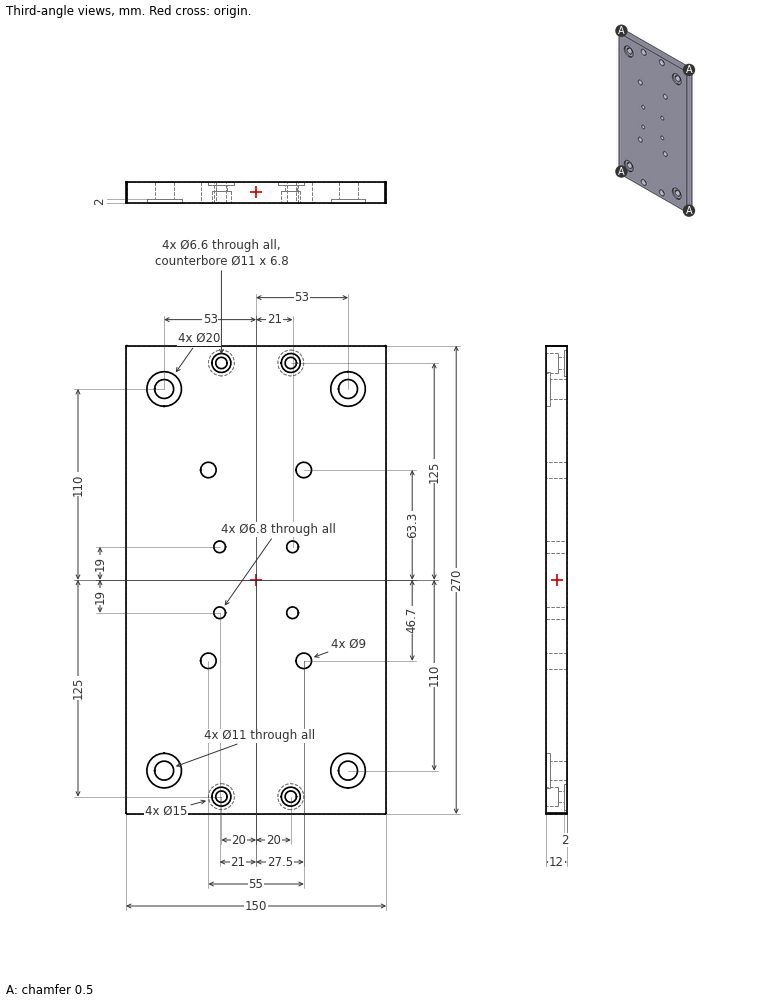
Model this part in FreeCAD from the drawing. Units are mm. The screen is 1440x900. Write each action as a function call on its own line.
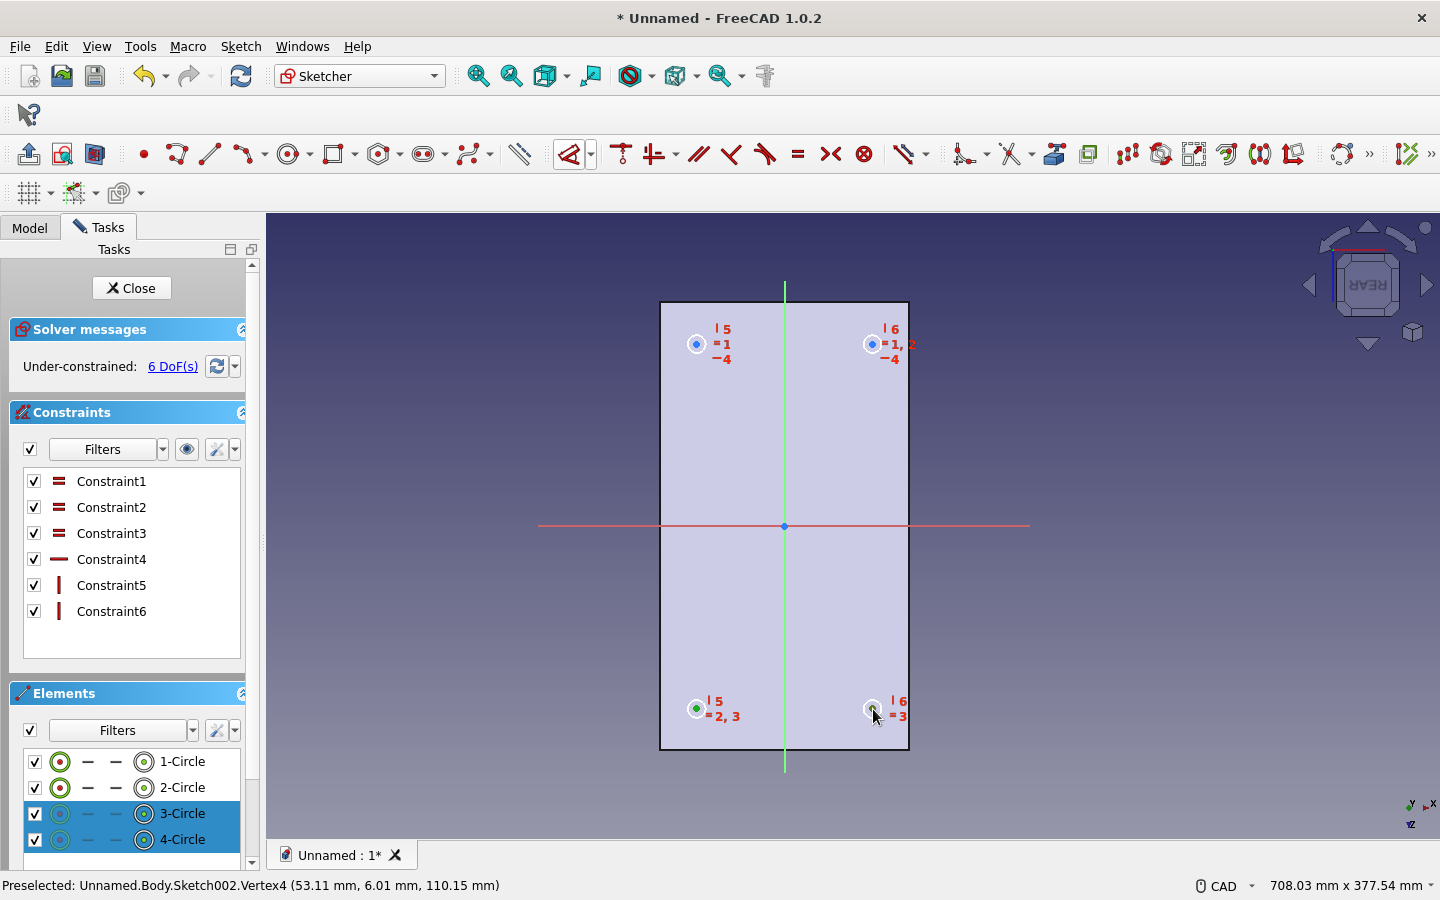
click(676, 154)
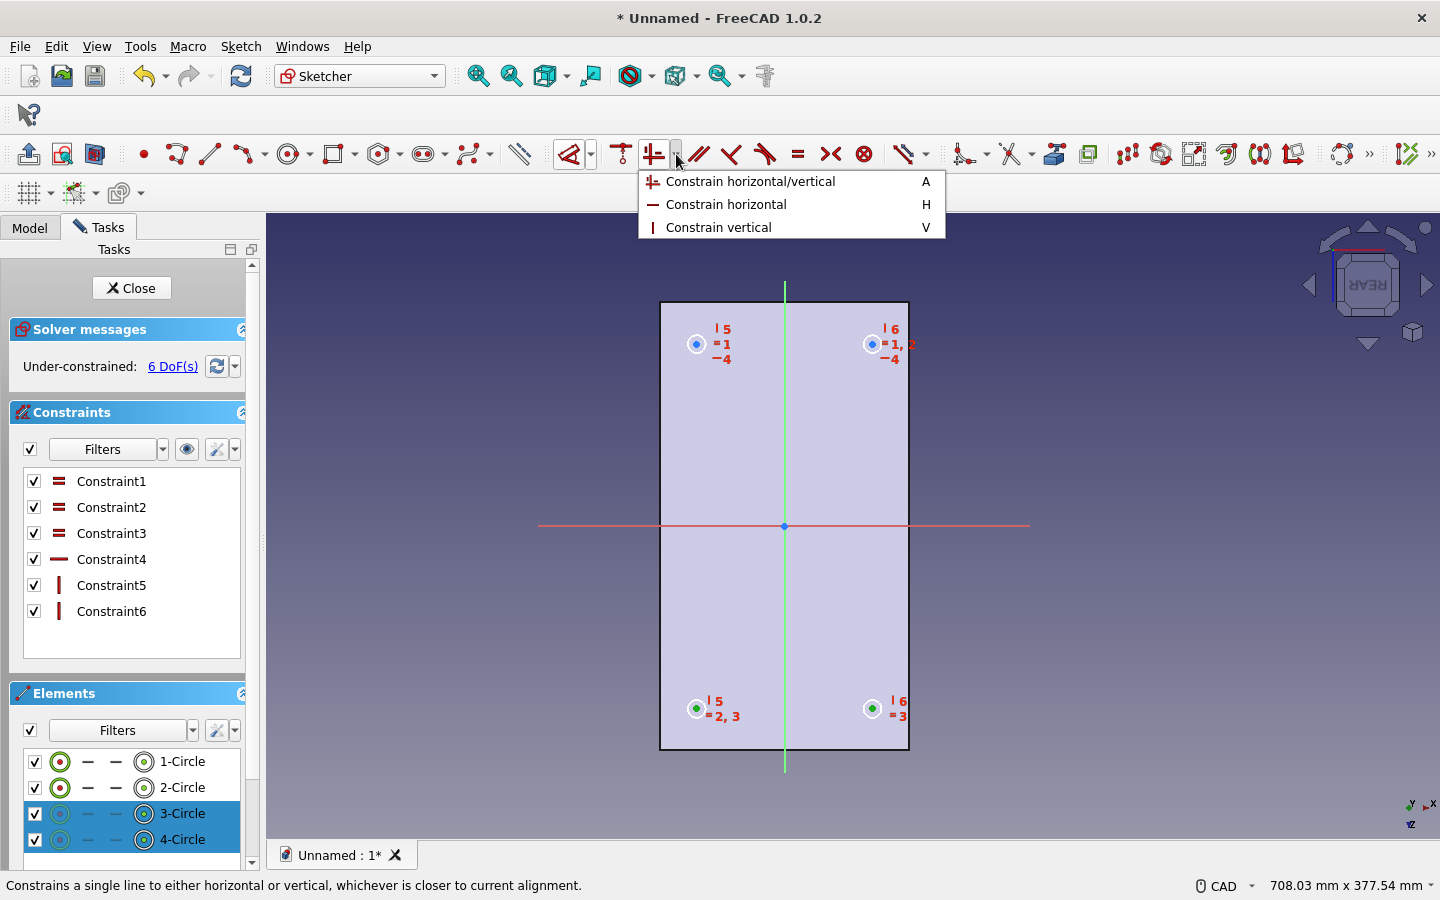
click(792, 204)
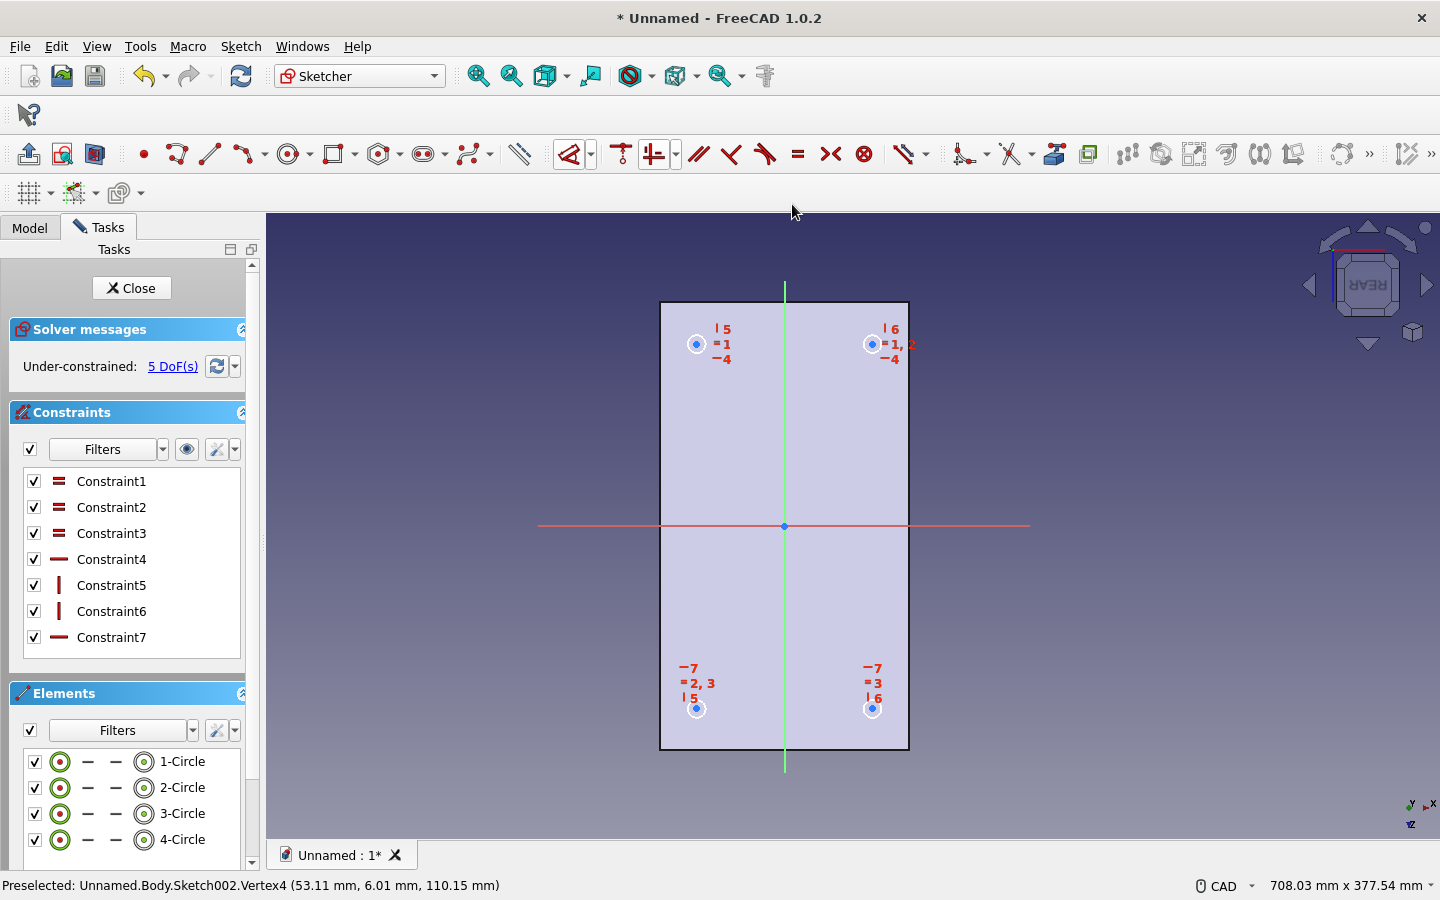
scroll(697, 335, up, 4)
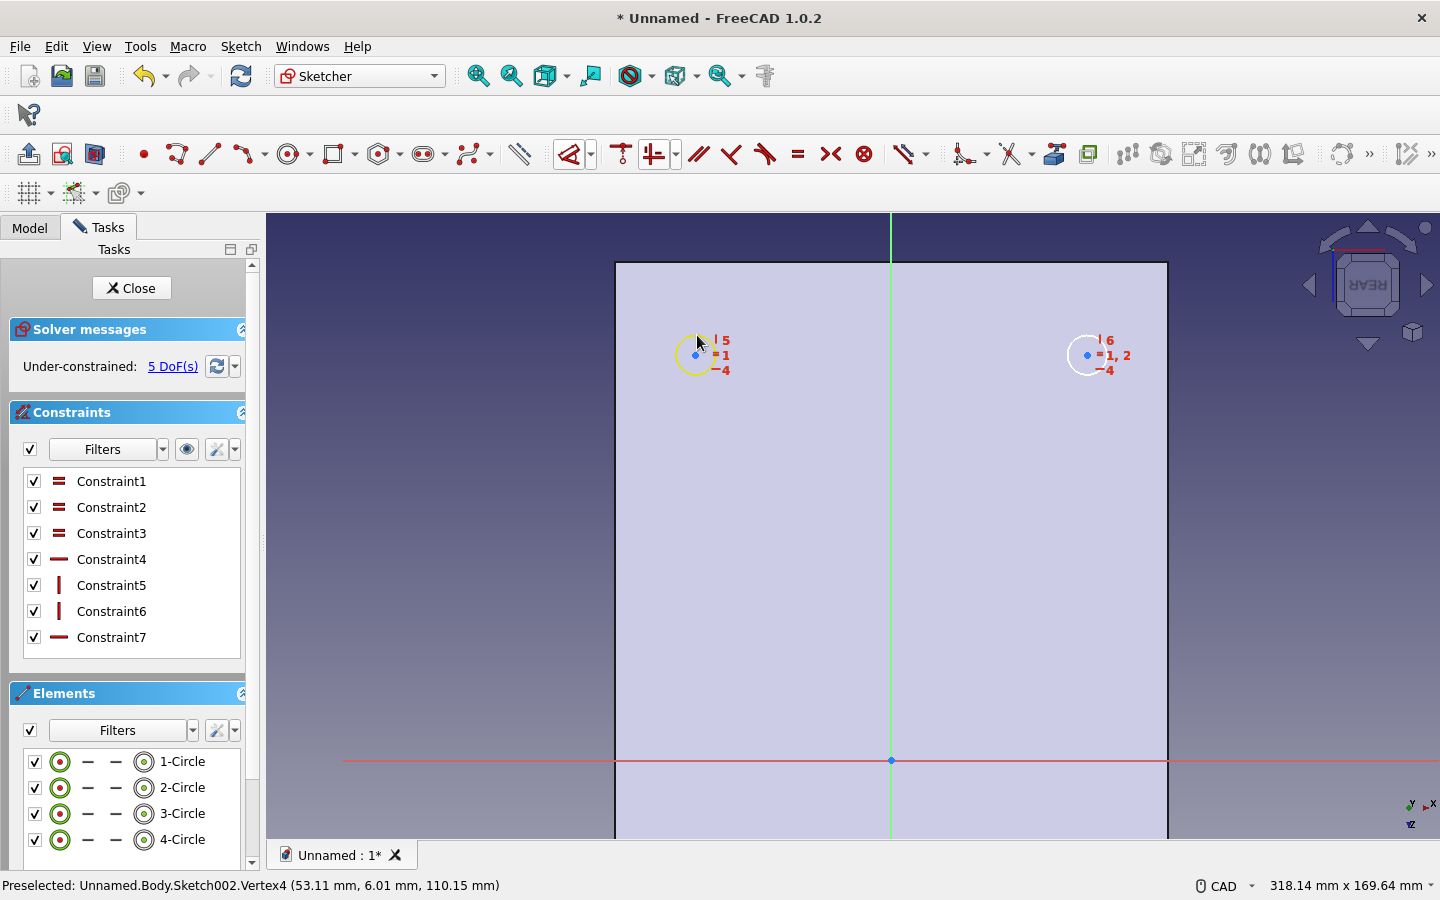
click(696, 335)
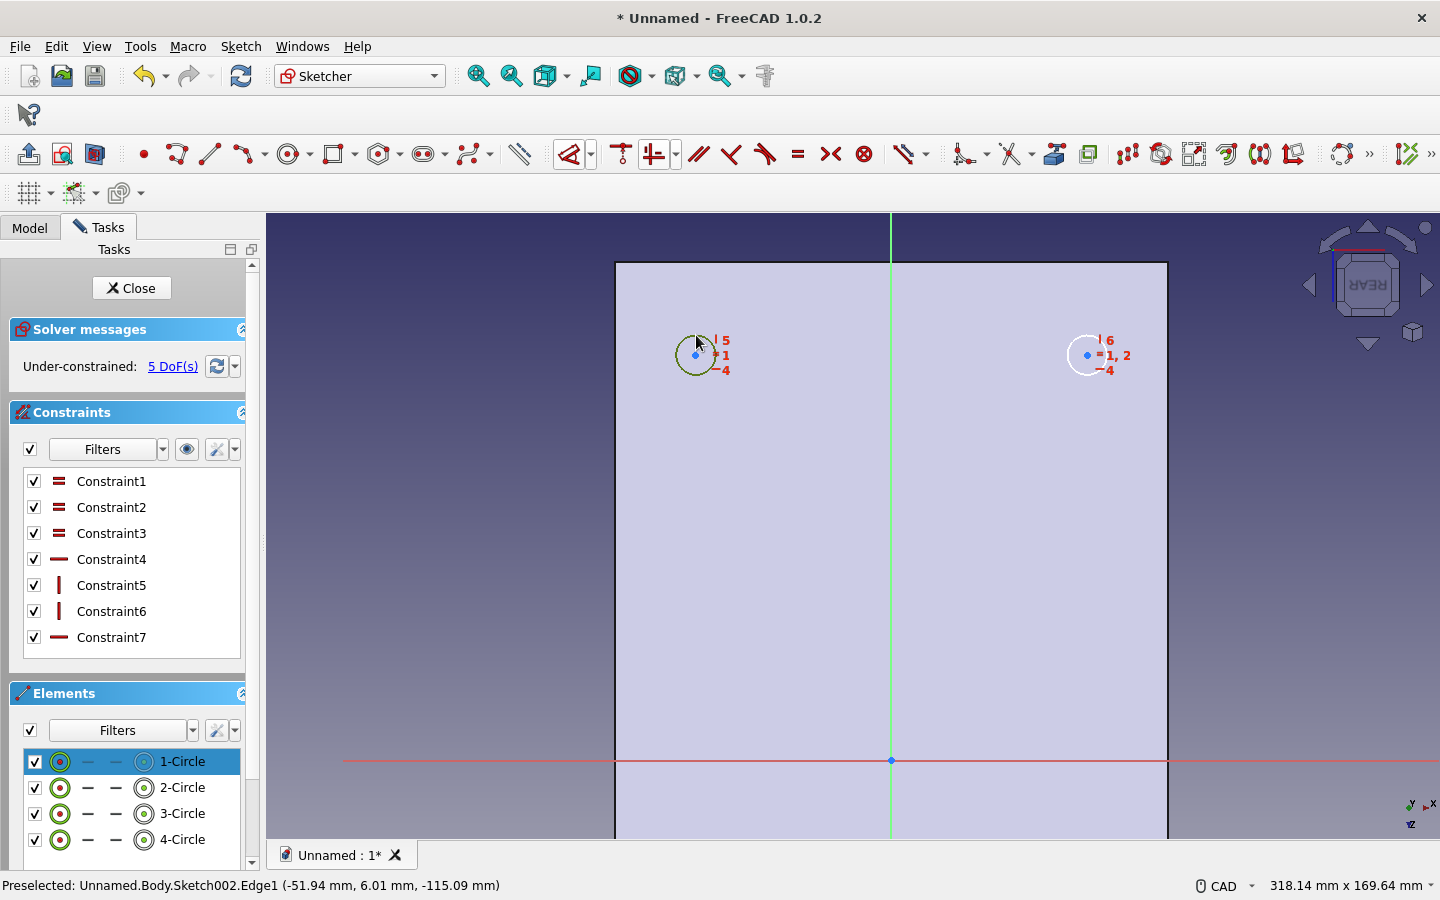
key(k)
key(o)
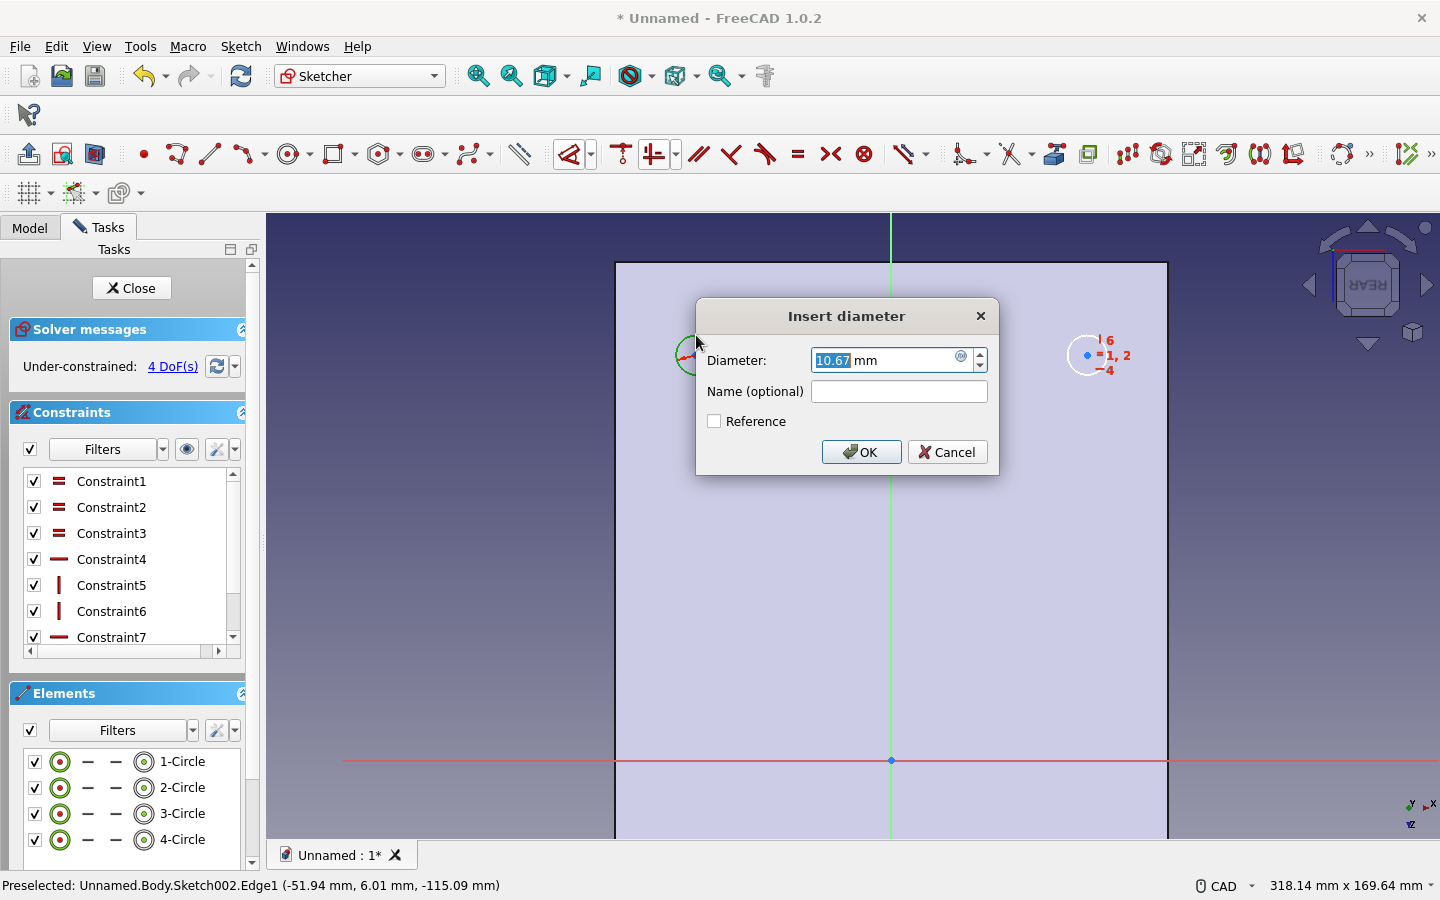
text(11)
key(Return)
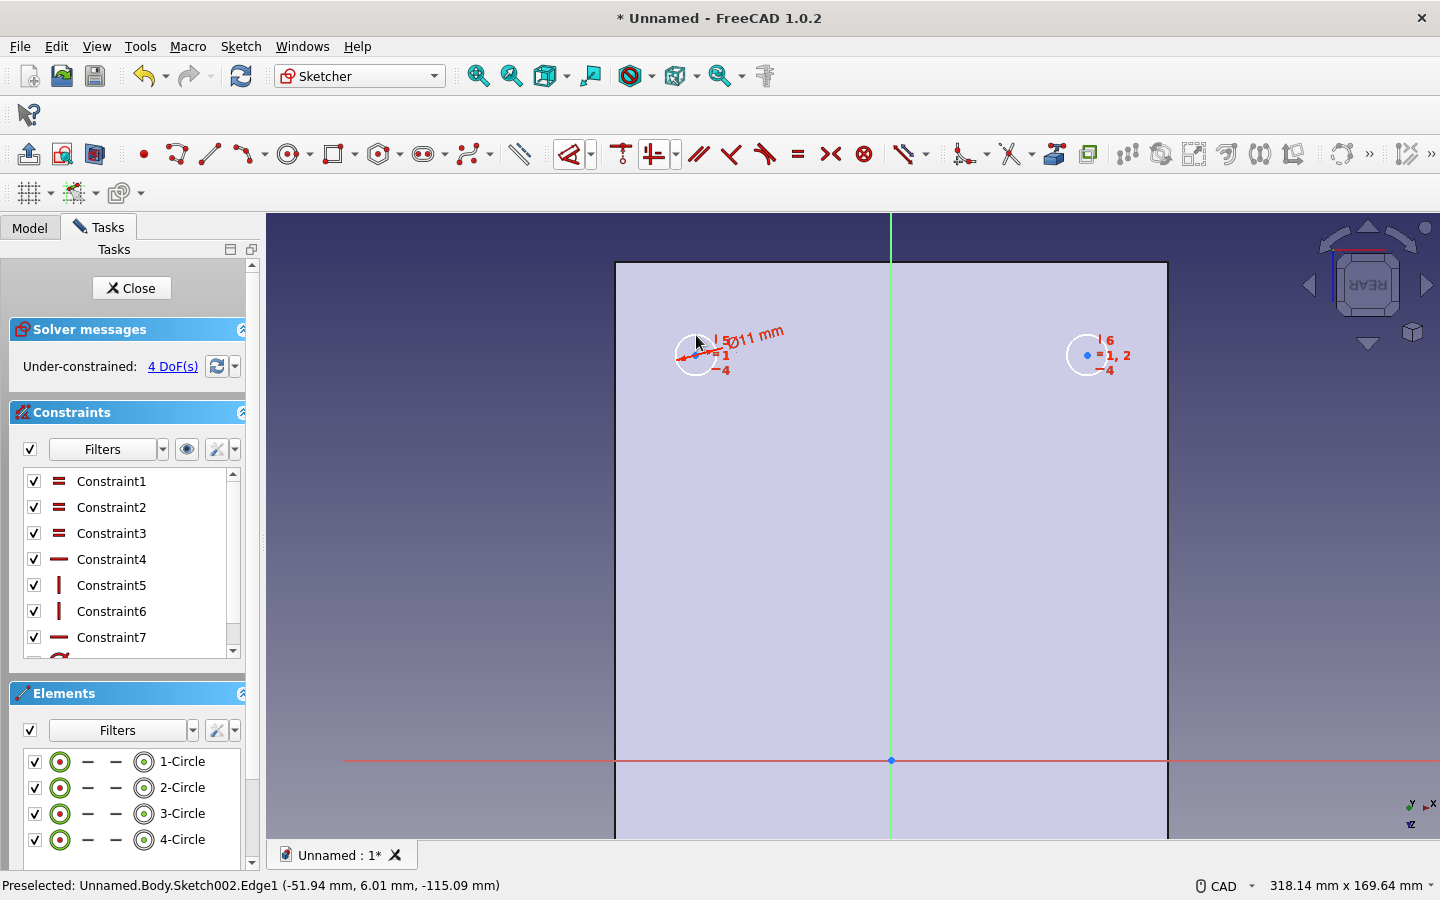
click(696, 355)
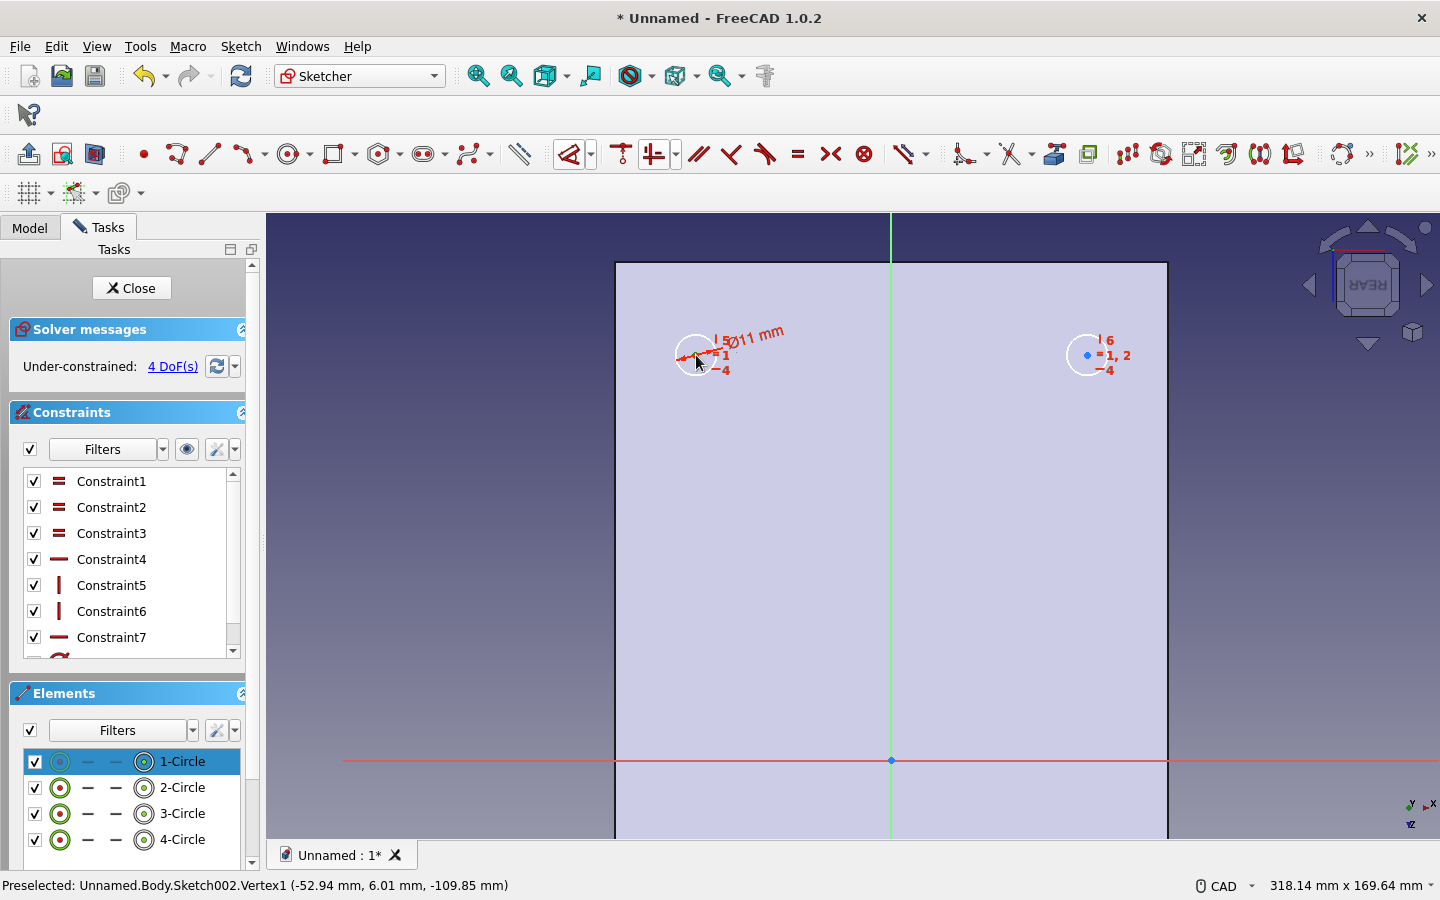
key(l)